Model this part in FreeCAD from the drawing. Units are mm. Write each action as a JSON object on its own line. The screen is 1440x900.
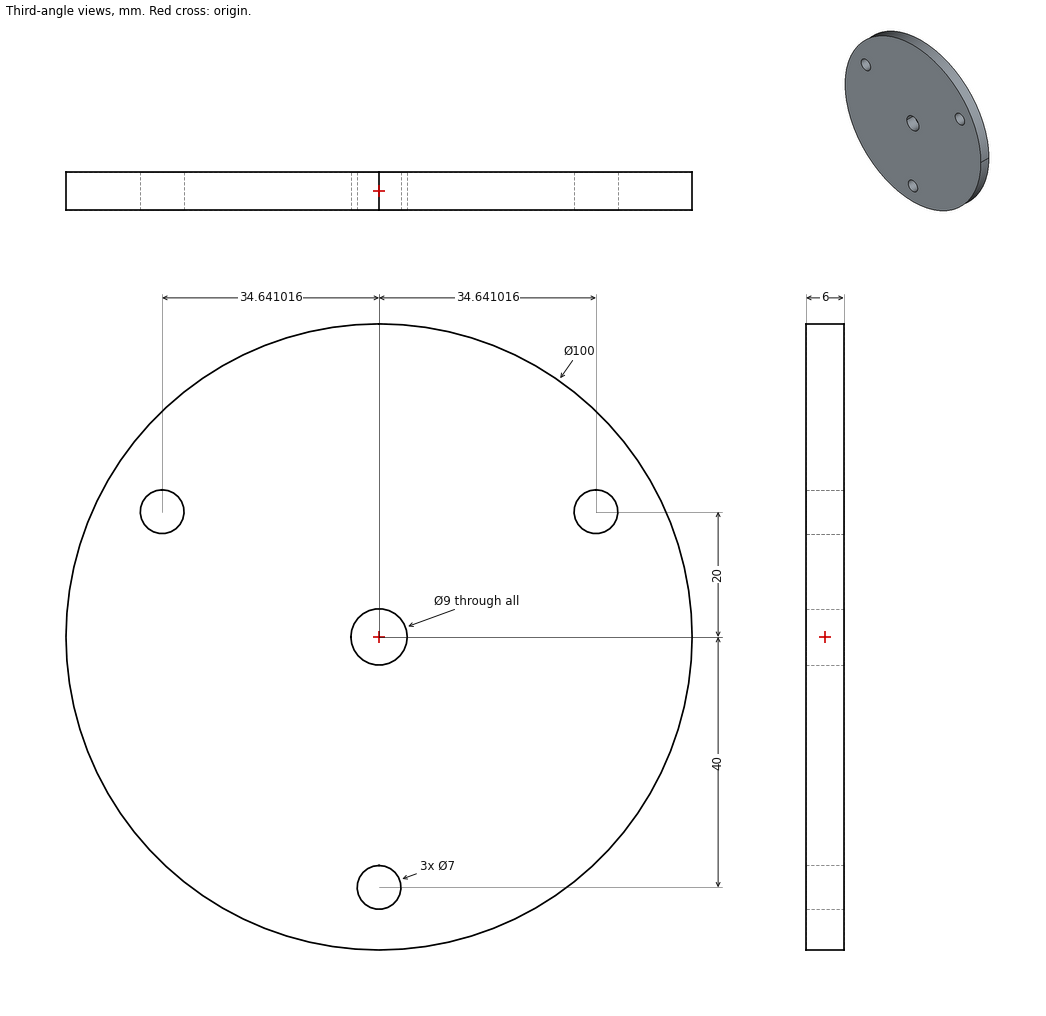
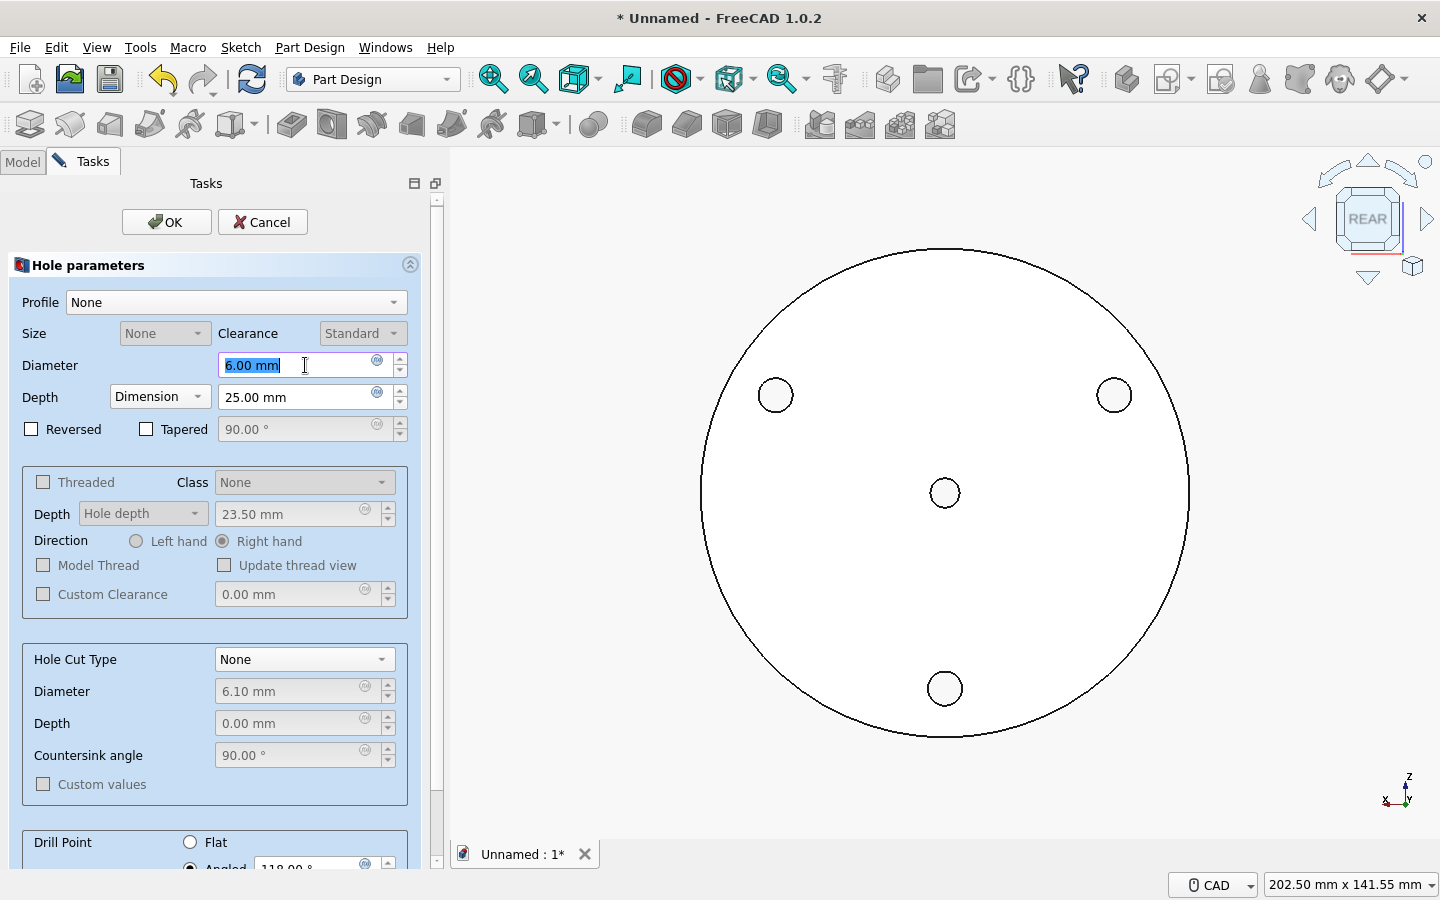
{"action": "type", "text": "9"}
{"action": "key", "text": "Tab"}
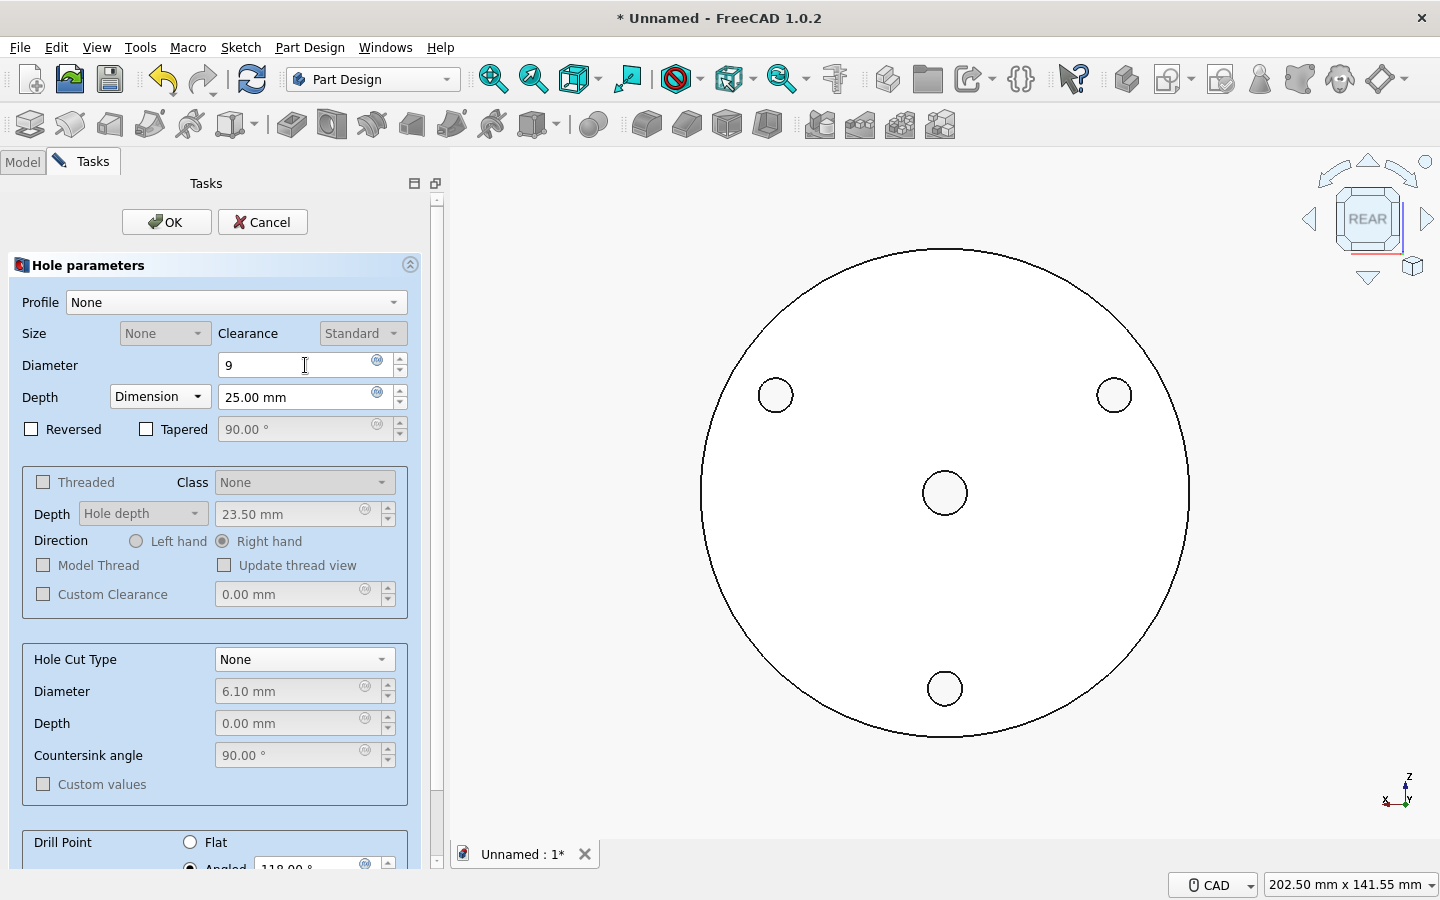
{"action": "left_click", "coordinate": [161, 396]}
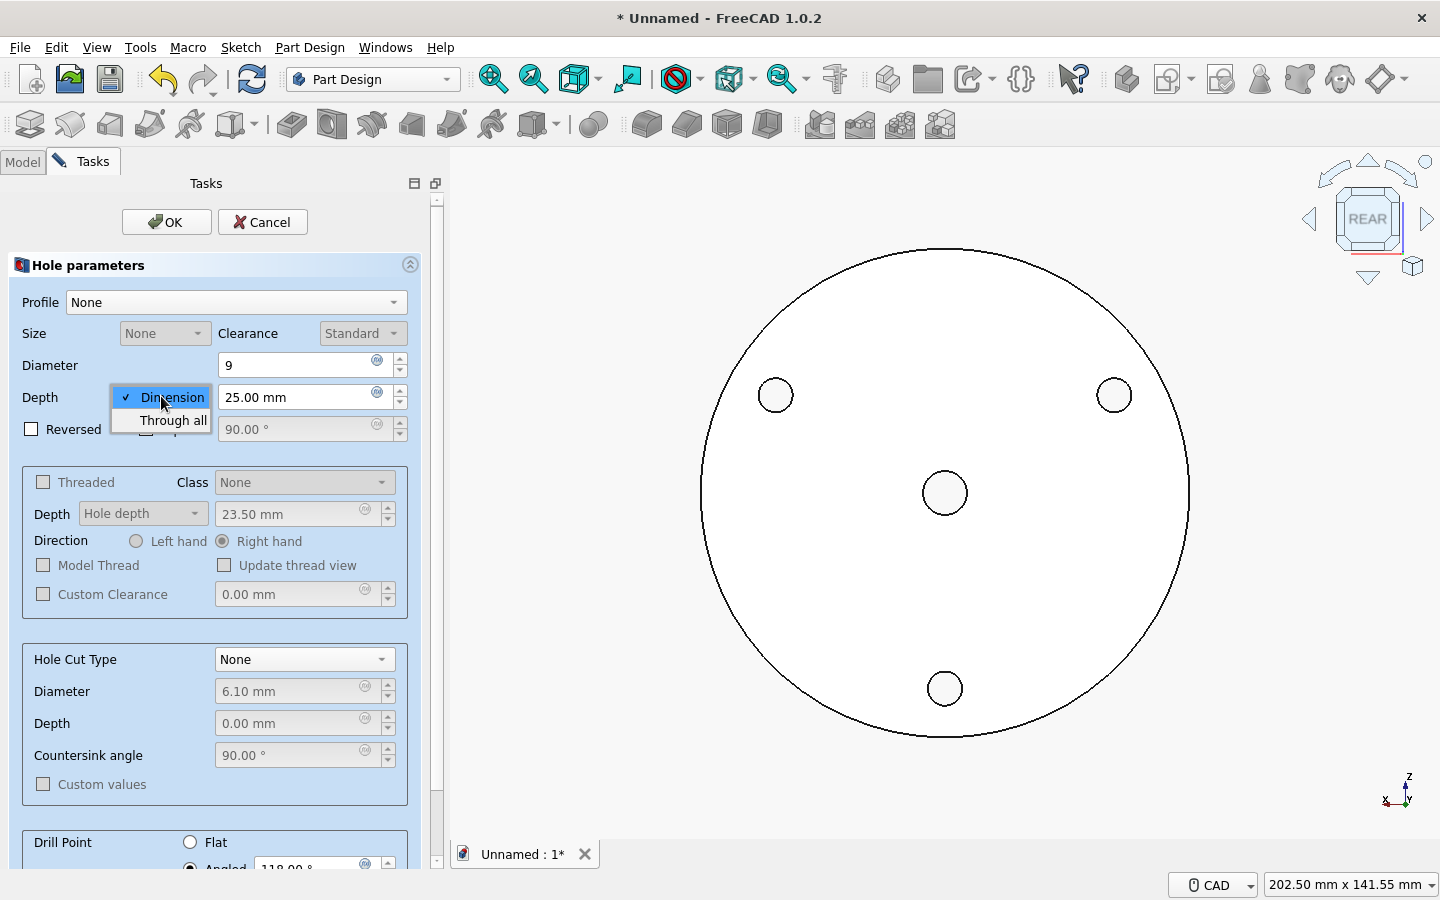
{"action": "left_click", "coordinate": [160, 420]}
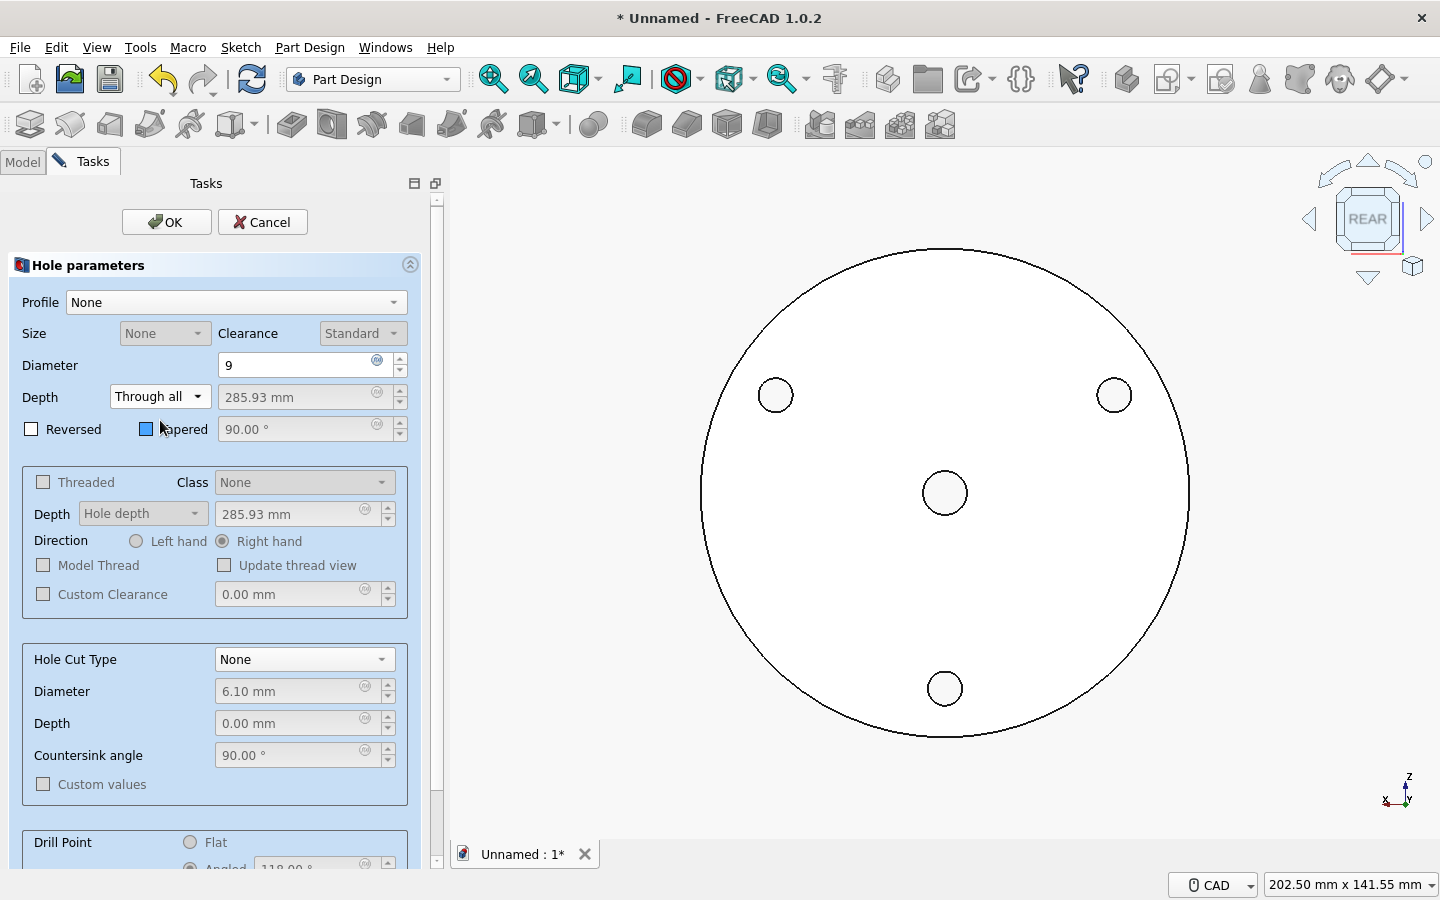
{"action": "left_click", "coordinate": [167, 222]}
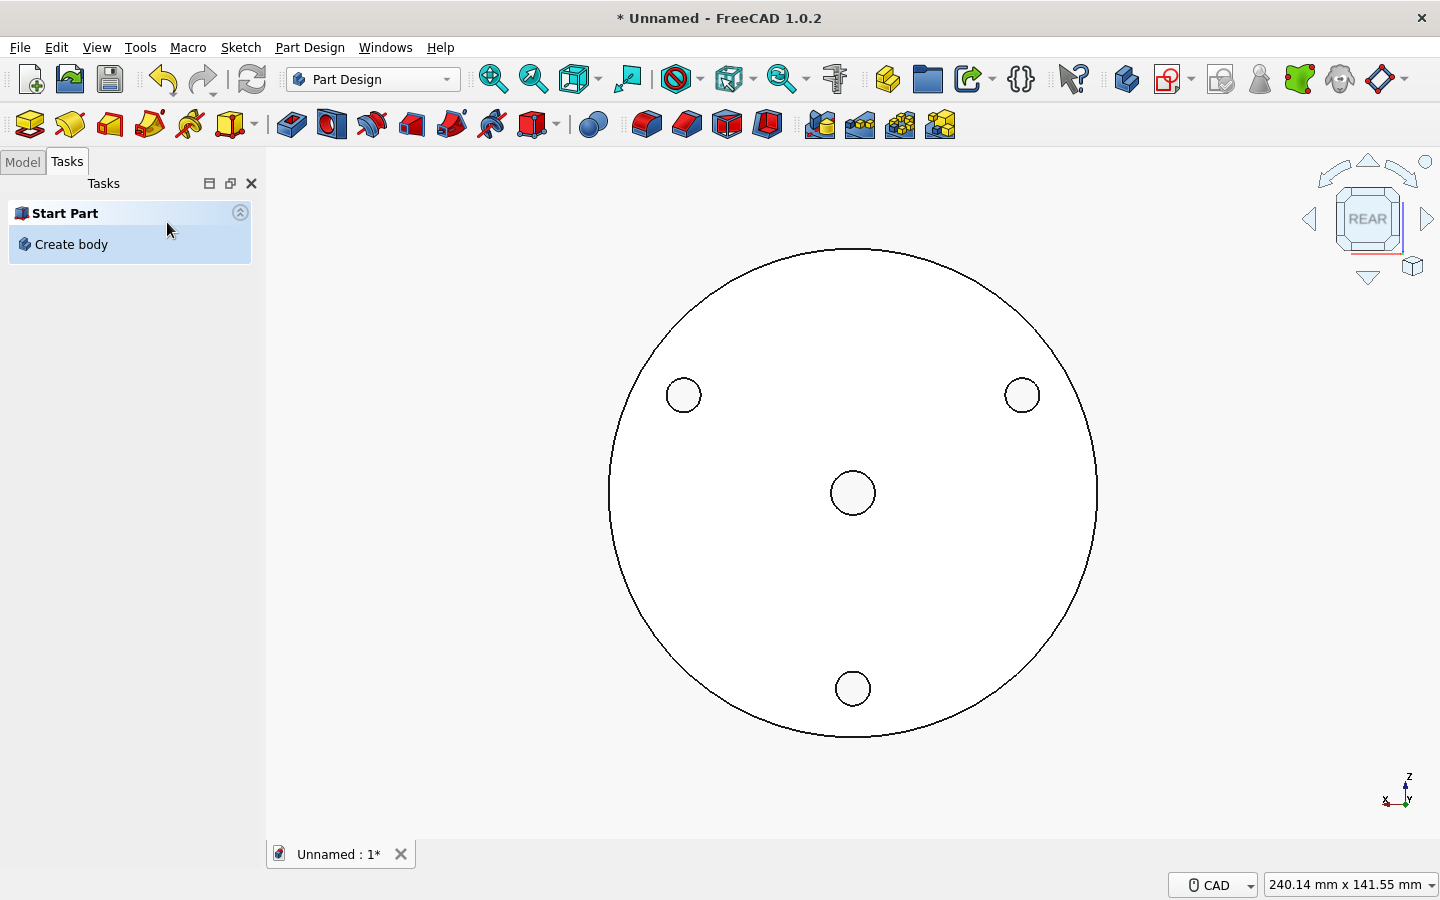
{"action": "key", "text": "0"}